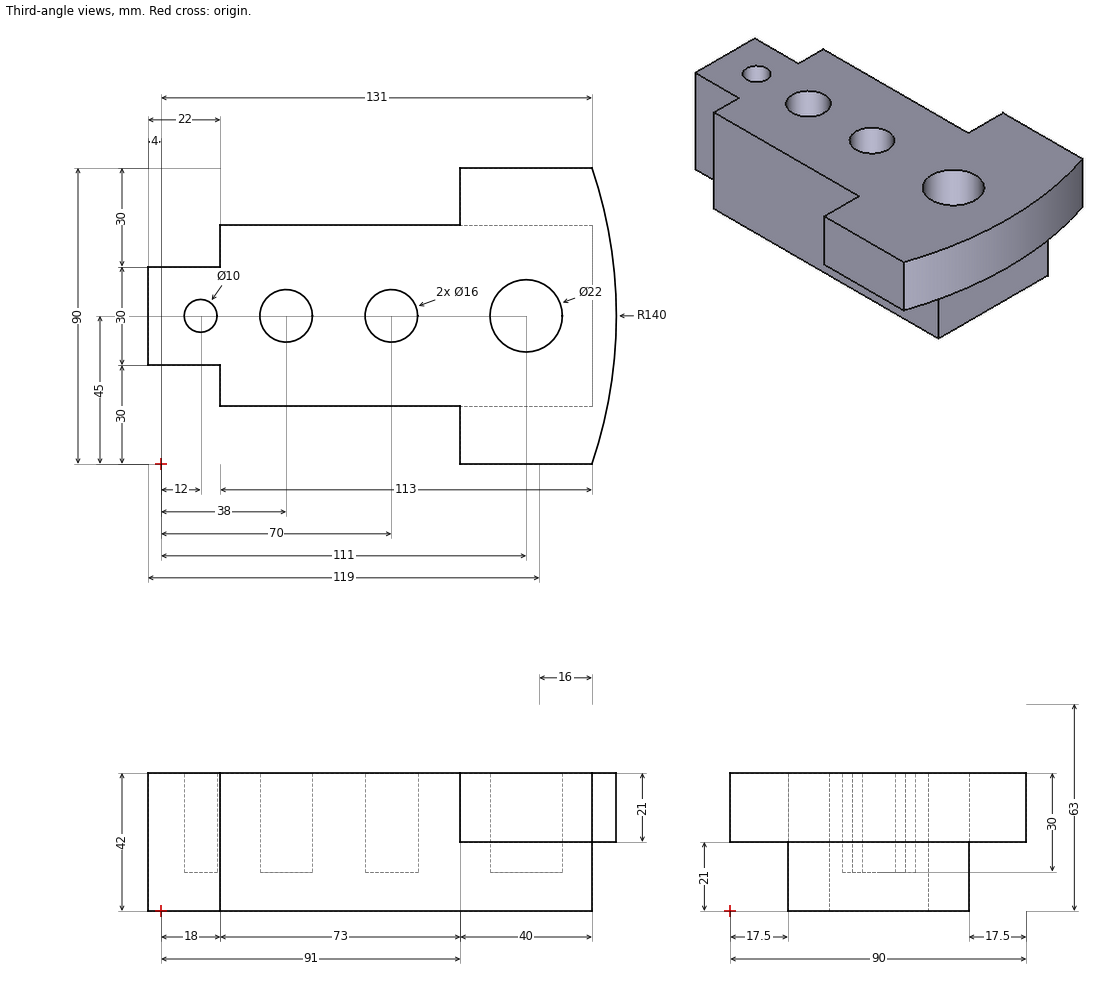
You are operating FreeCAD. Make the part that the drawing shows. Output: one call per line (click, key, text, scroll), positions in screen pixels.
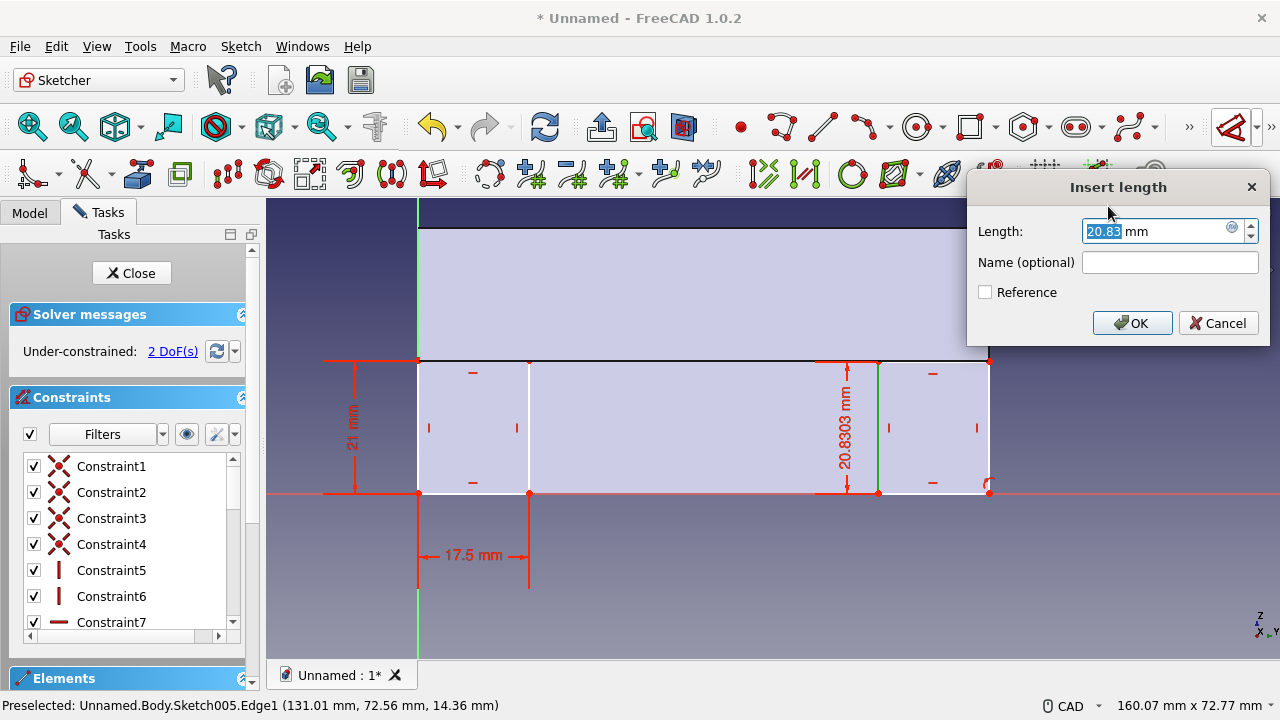
text(21)
key(Return)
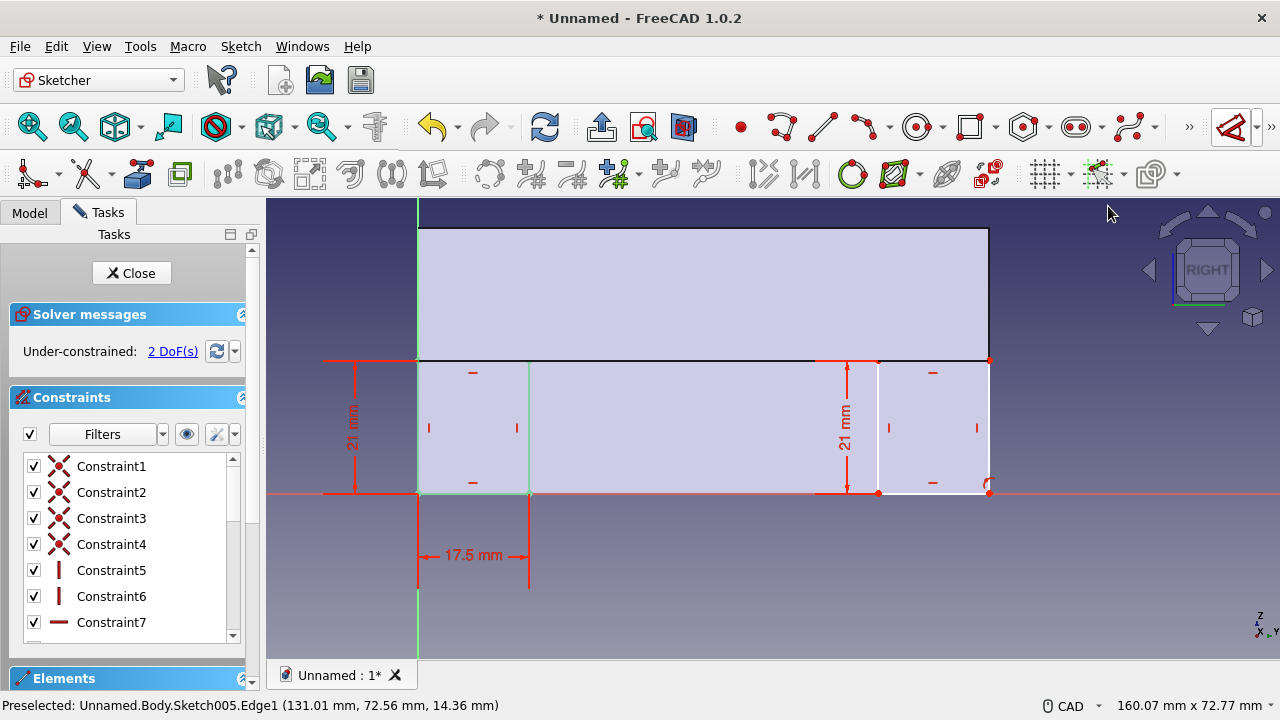
click(989, 494)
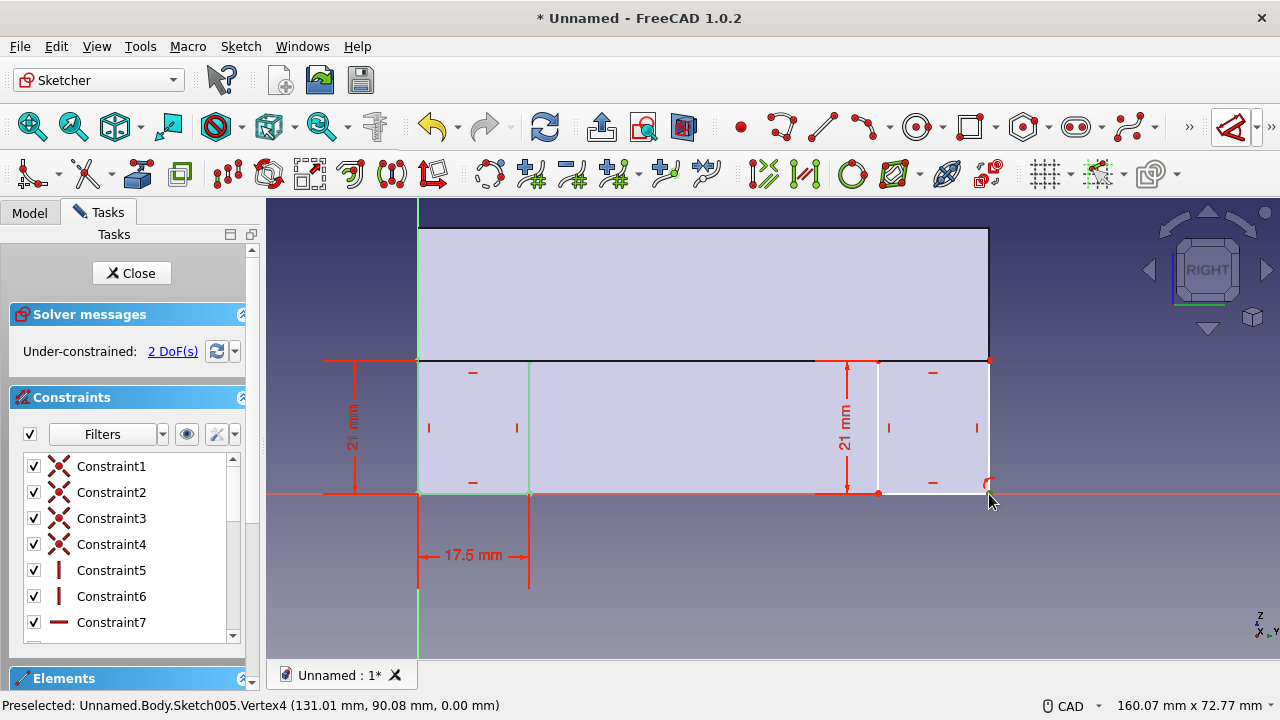
click(1256, 128)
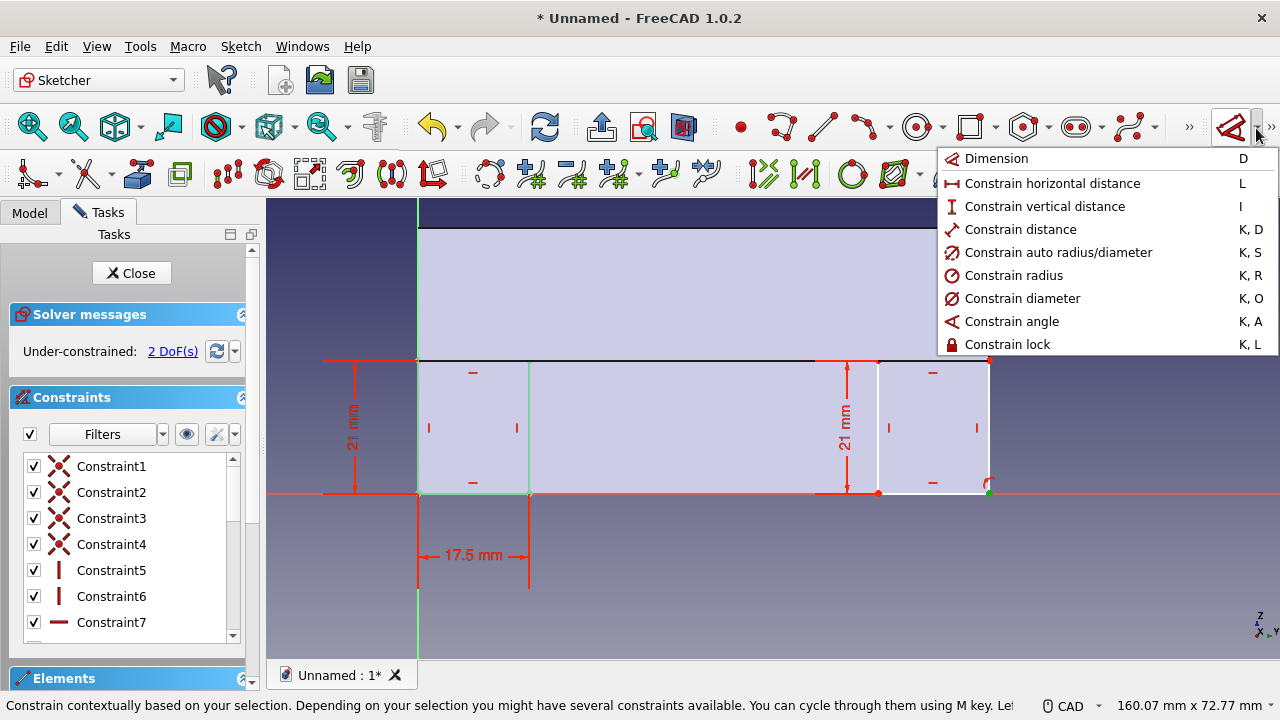
click(1108, 184)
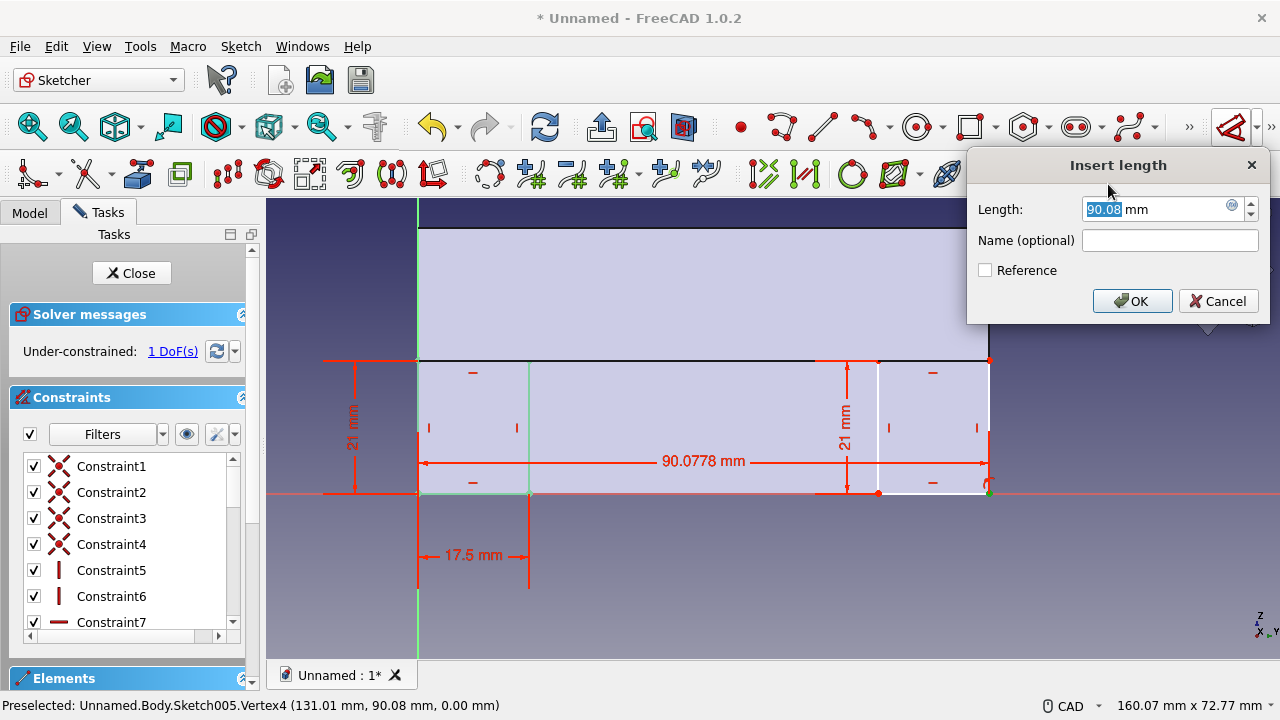
text(90)
key(Return)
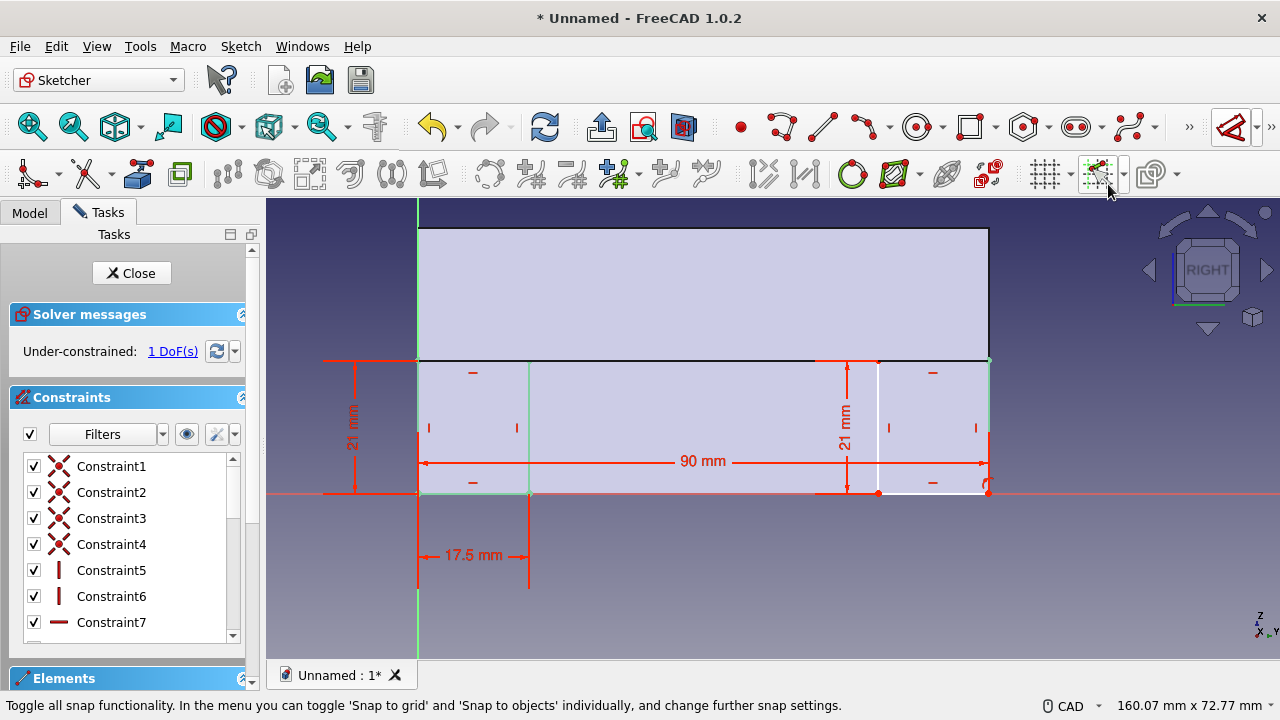
click(911, 494)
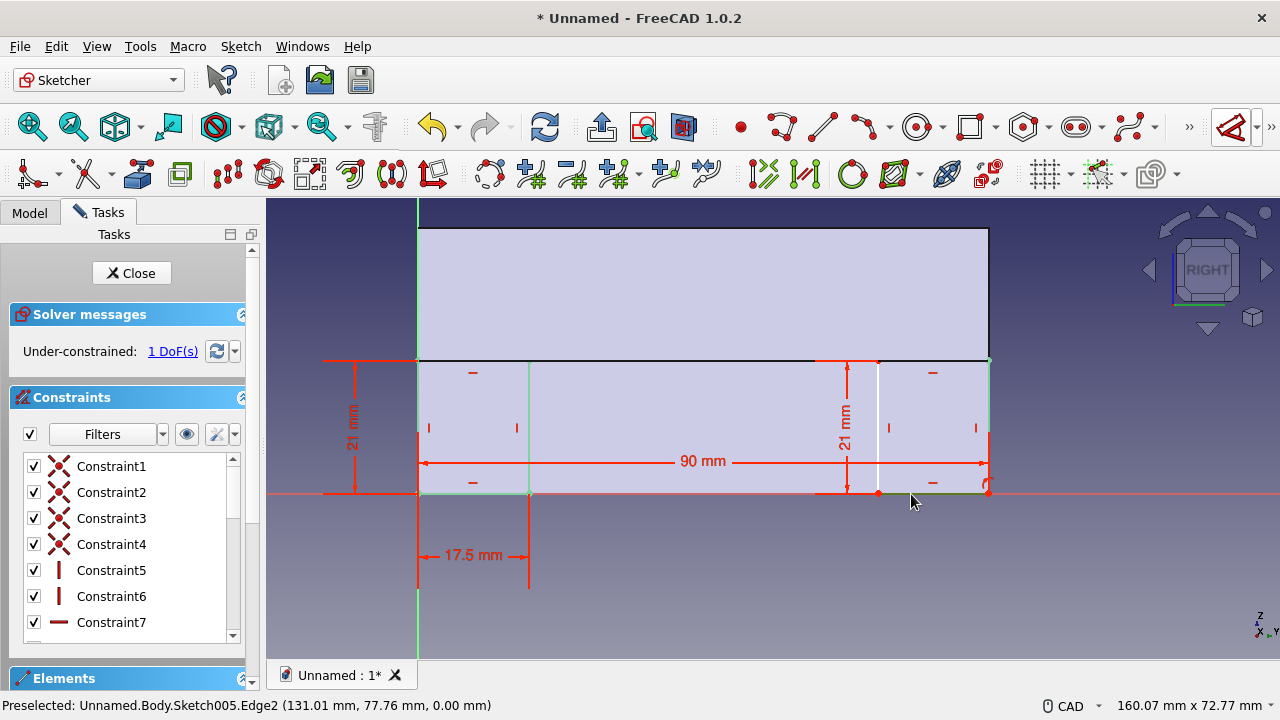
key(l)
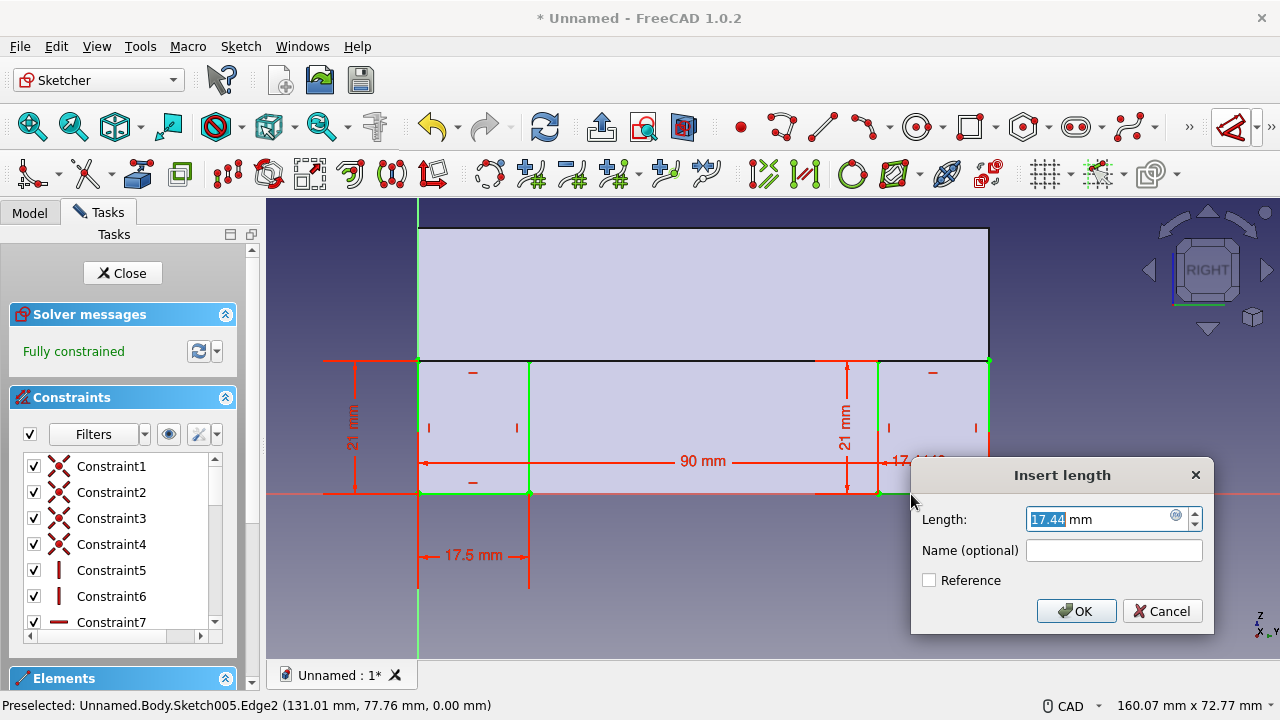
text(17.5)
key(Return)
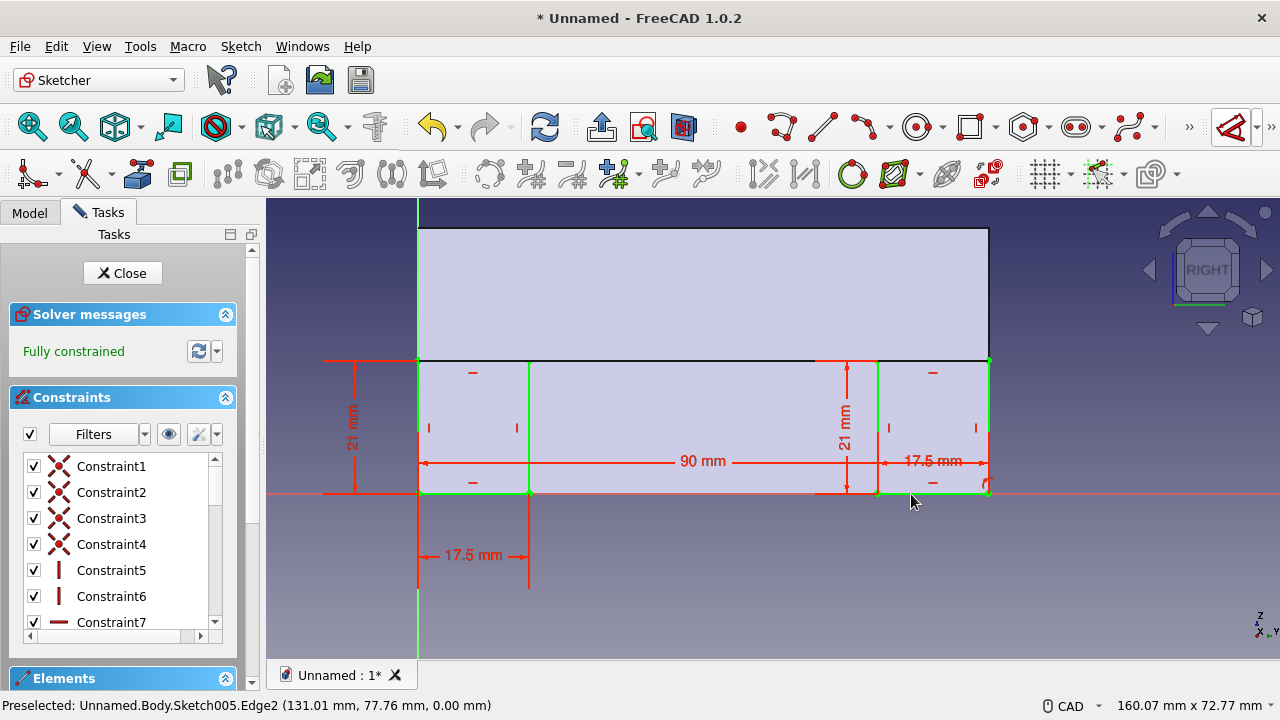
click(123, 273)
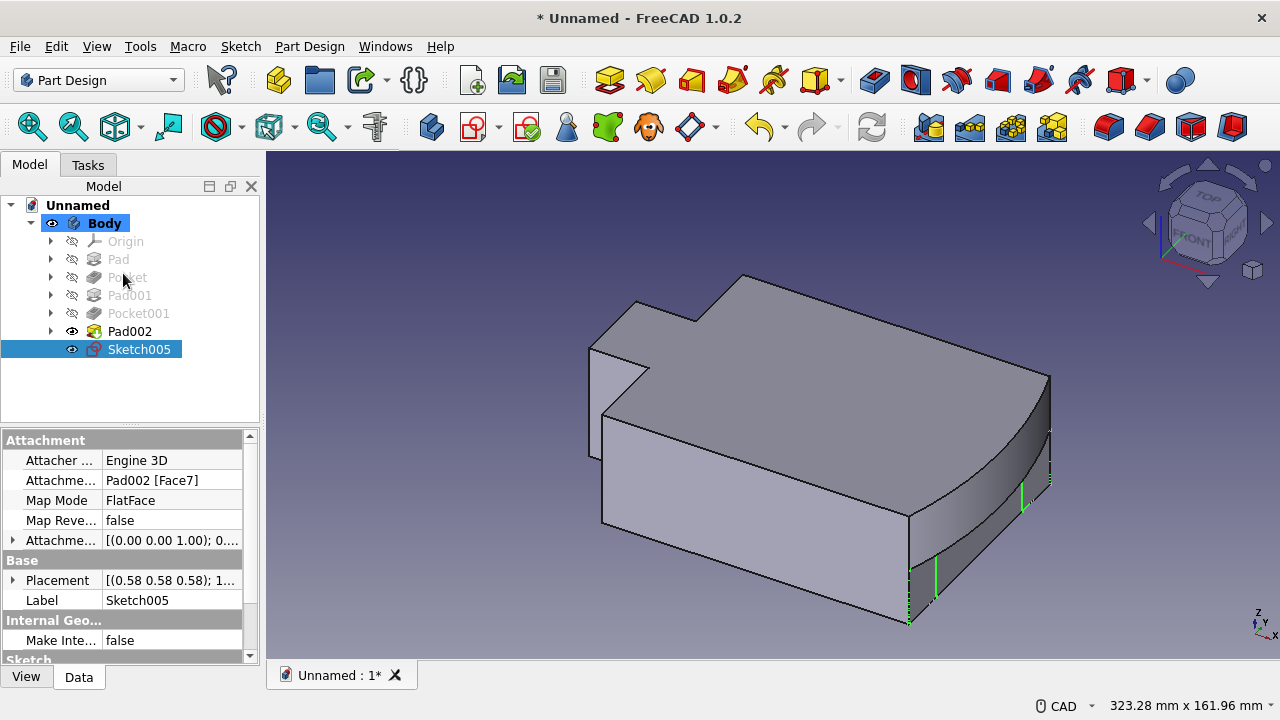
click(875, 80)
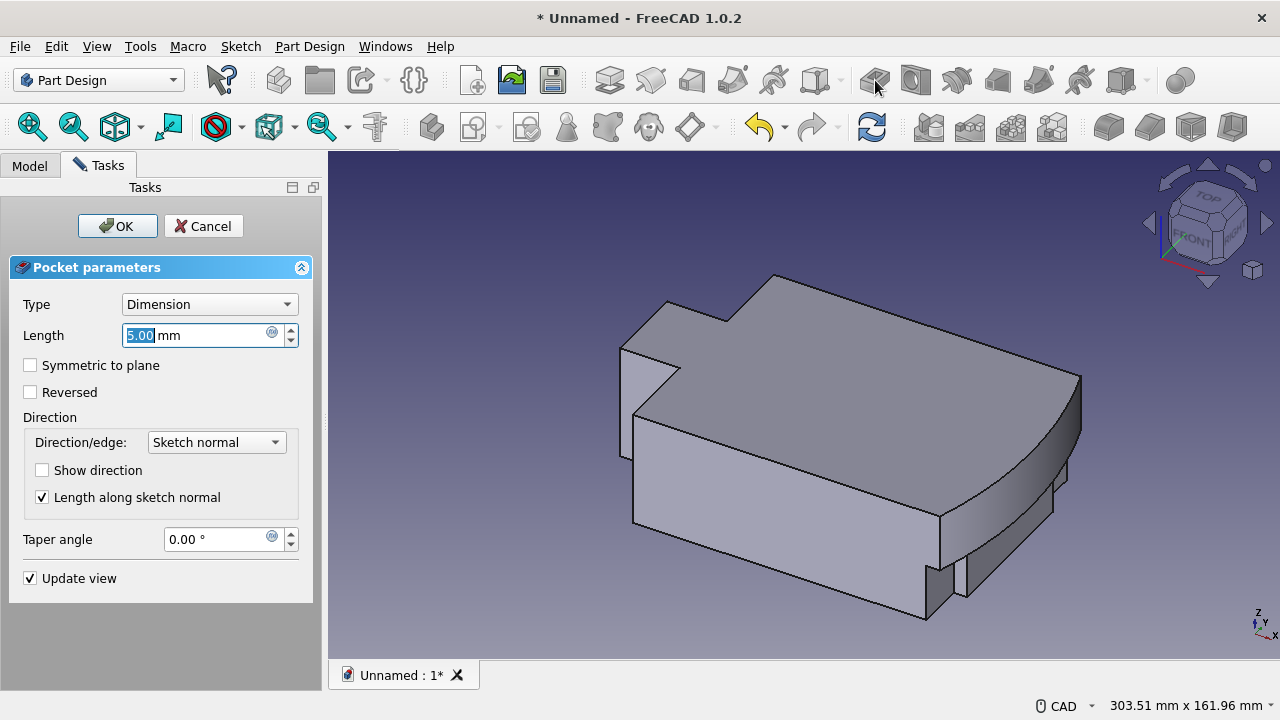
text(40)
key(Tab)